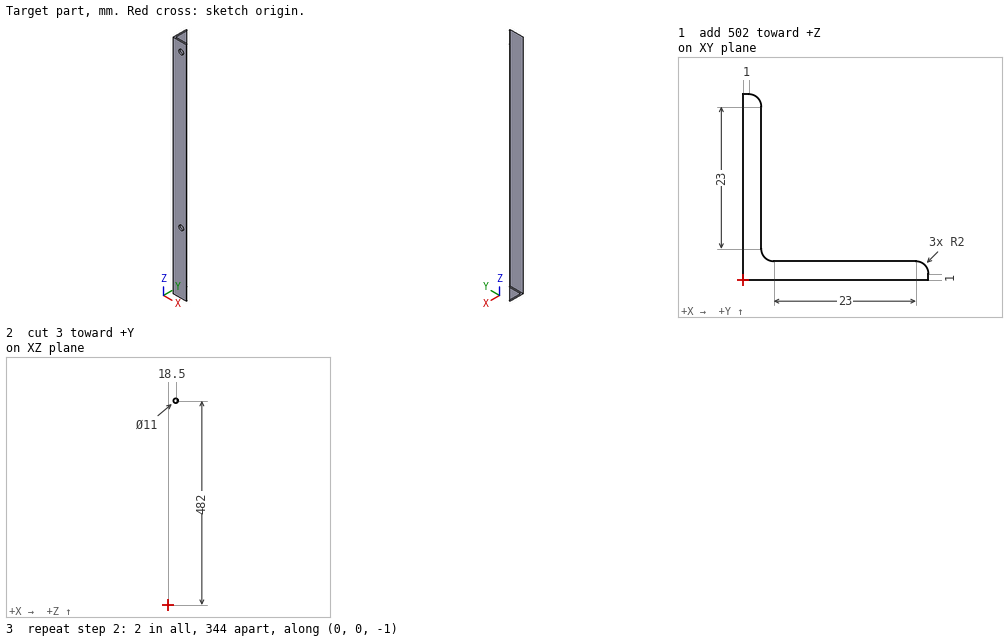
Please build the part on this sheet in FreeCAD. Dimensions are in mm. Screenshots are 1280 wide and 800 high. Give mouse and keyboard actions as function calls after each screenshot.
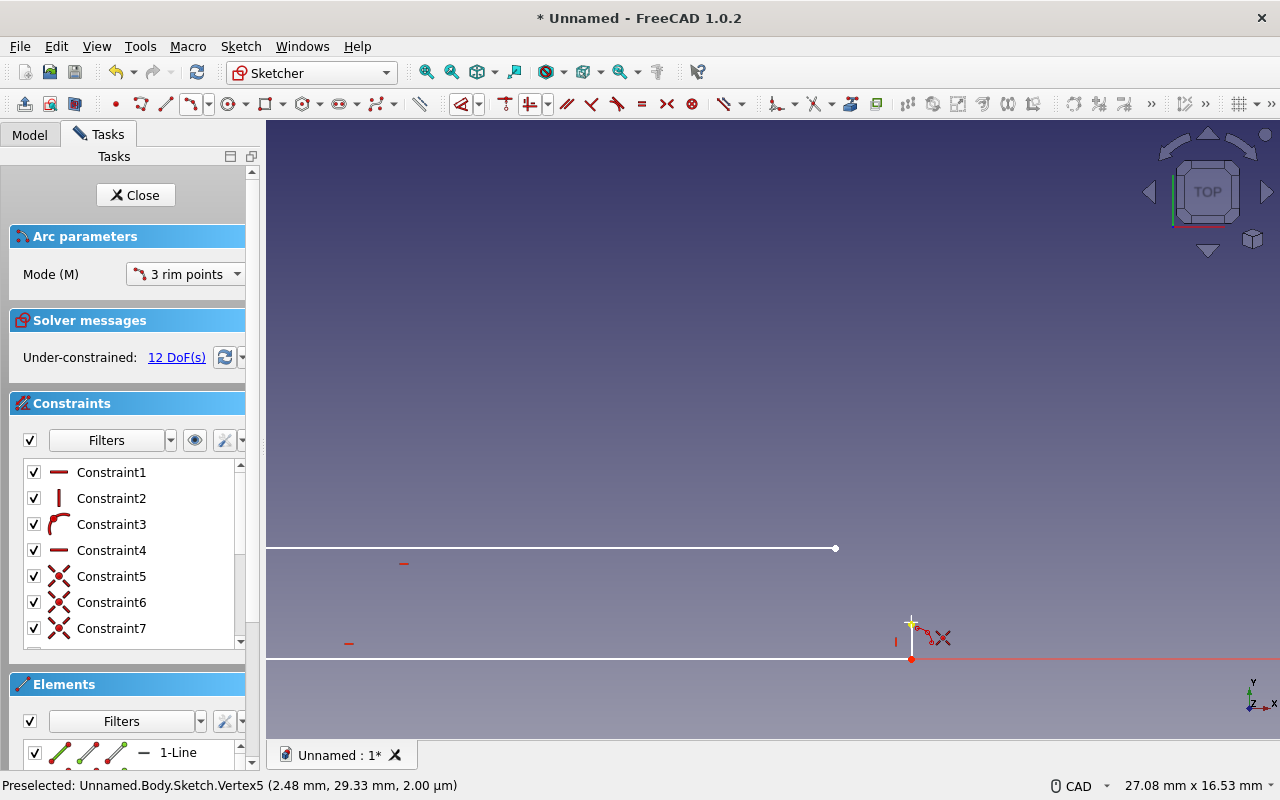
click(912, 625)
click(836, 548)
click(889, 569)
key(Escape)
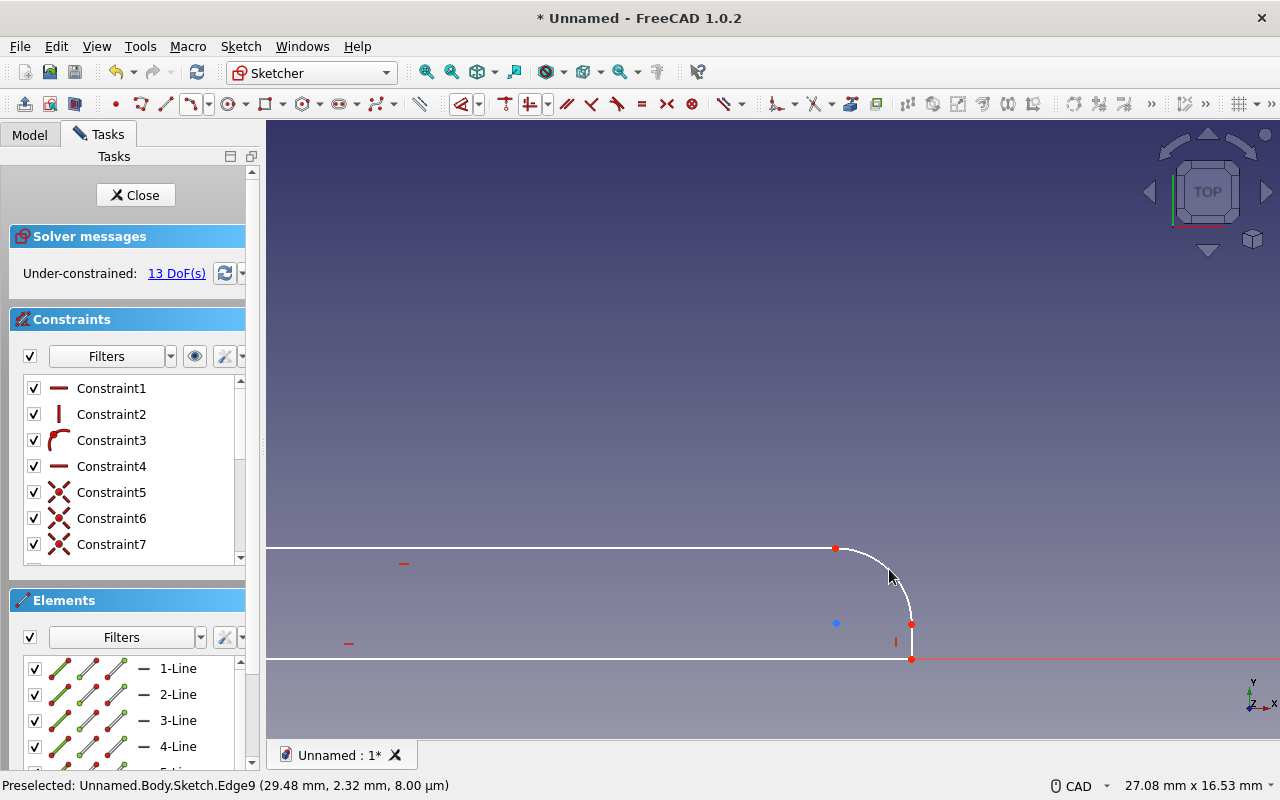
click(577, 548)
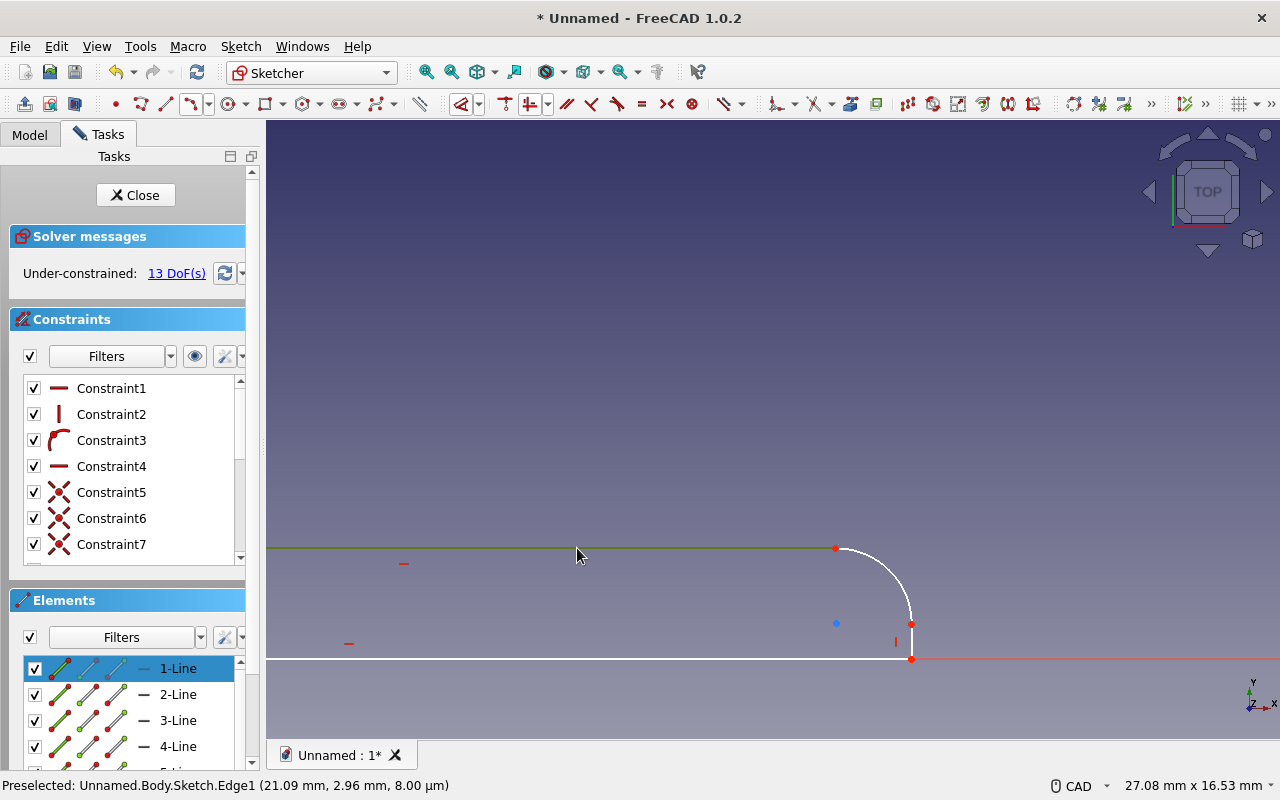
scroll(911, 623, down, 5)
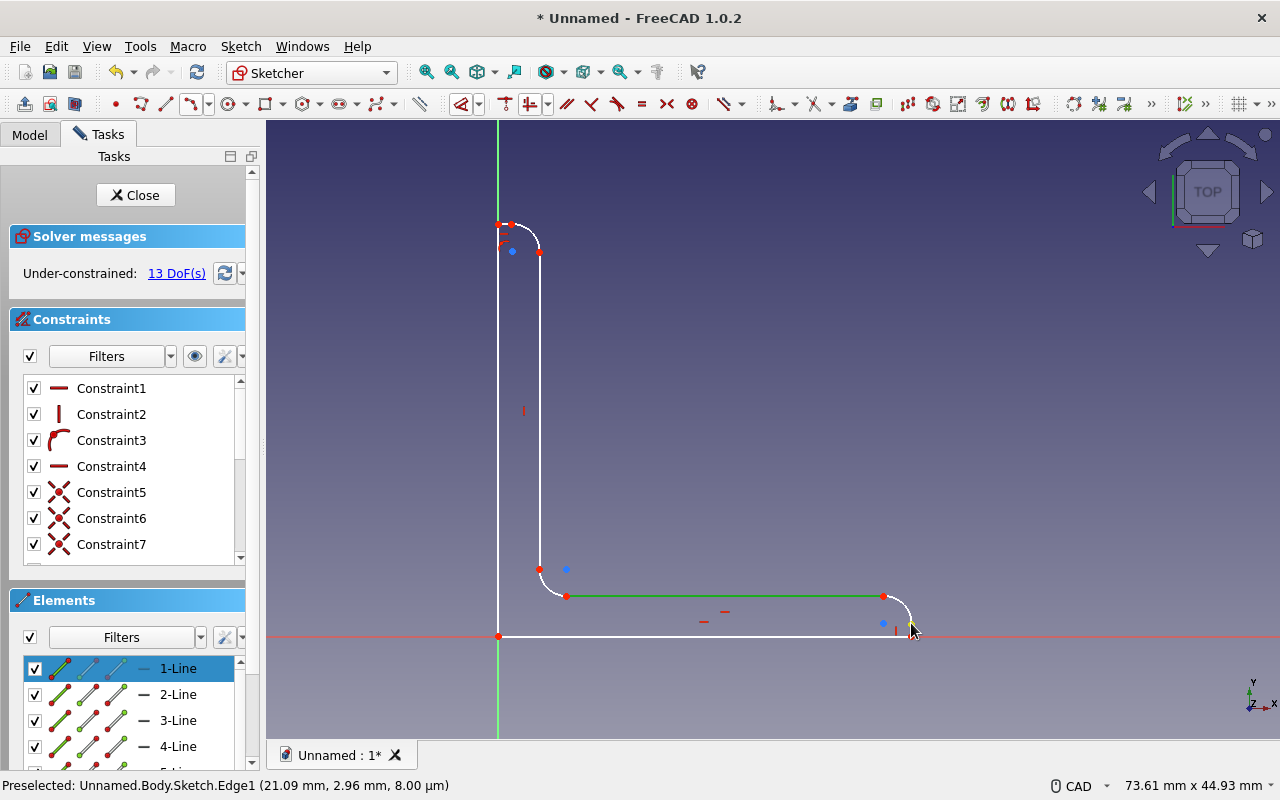
click(543, 581)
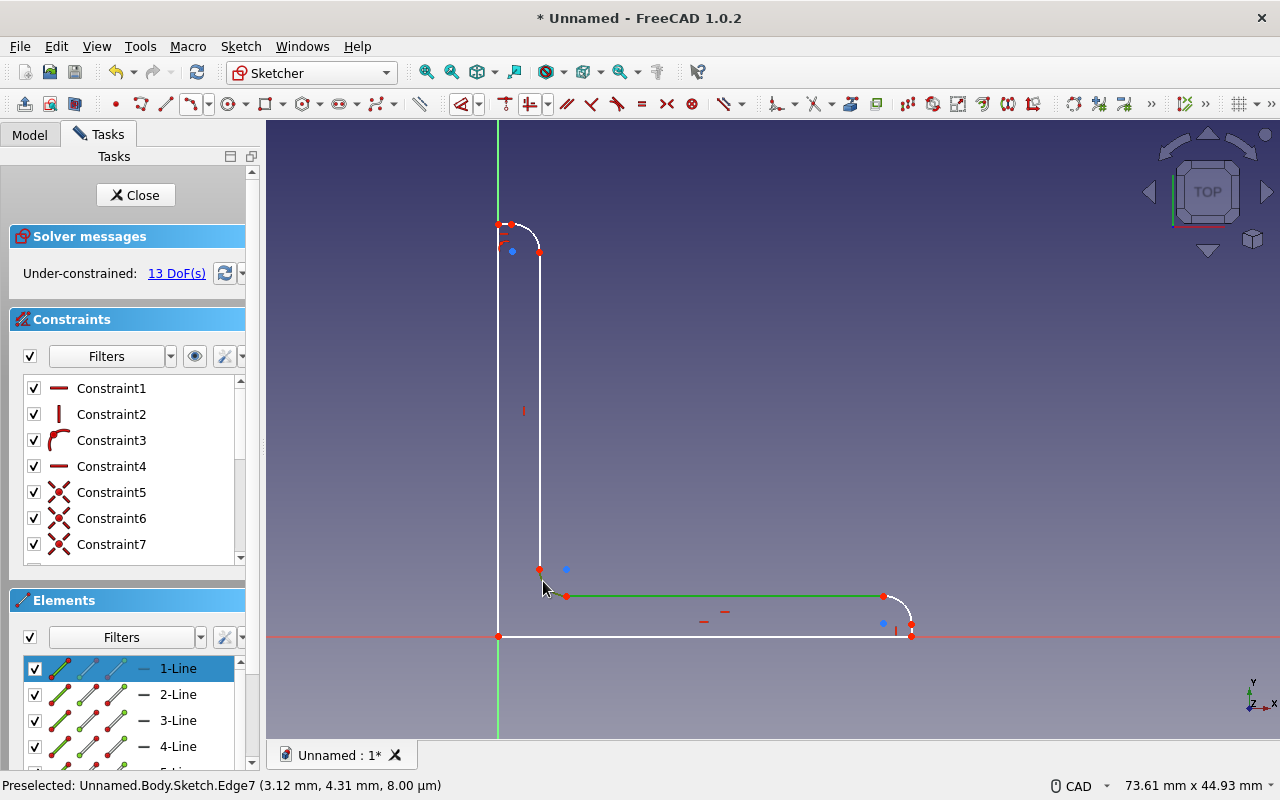
click(617, 104)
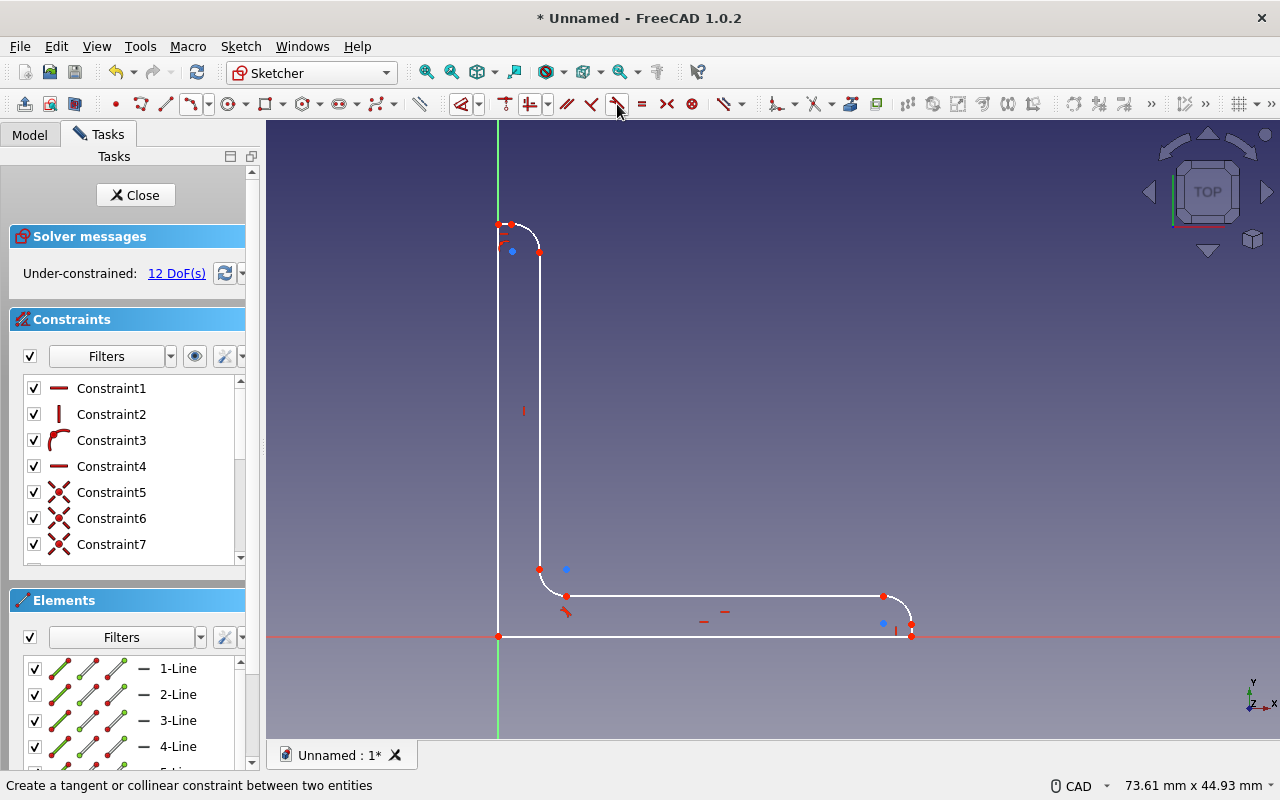
click(789, 596)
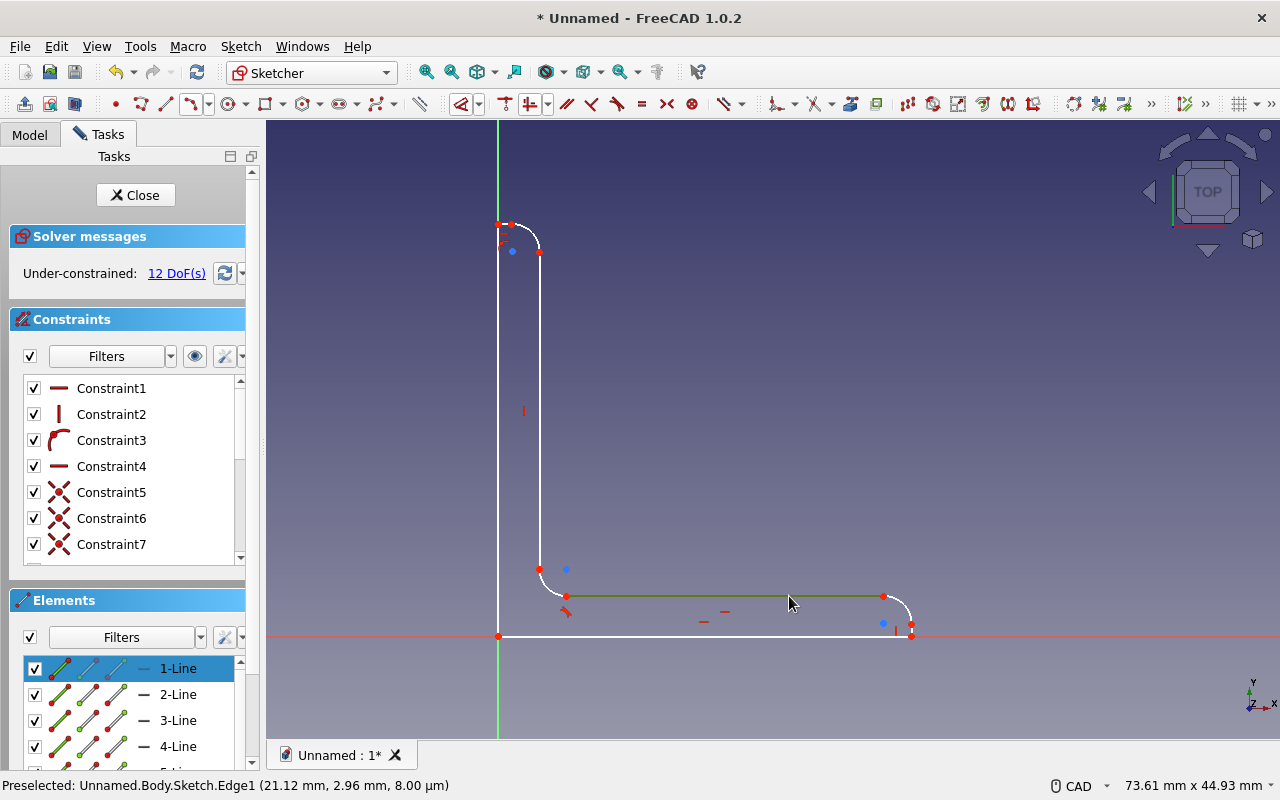
click(909, 611)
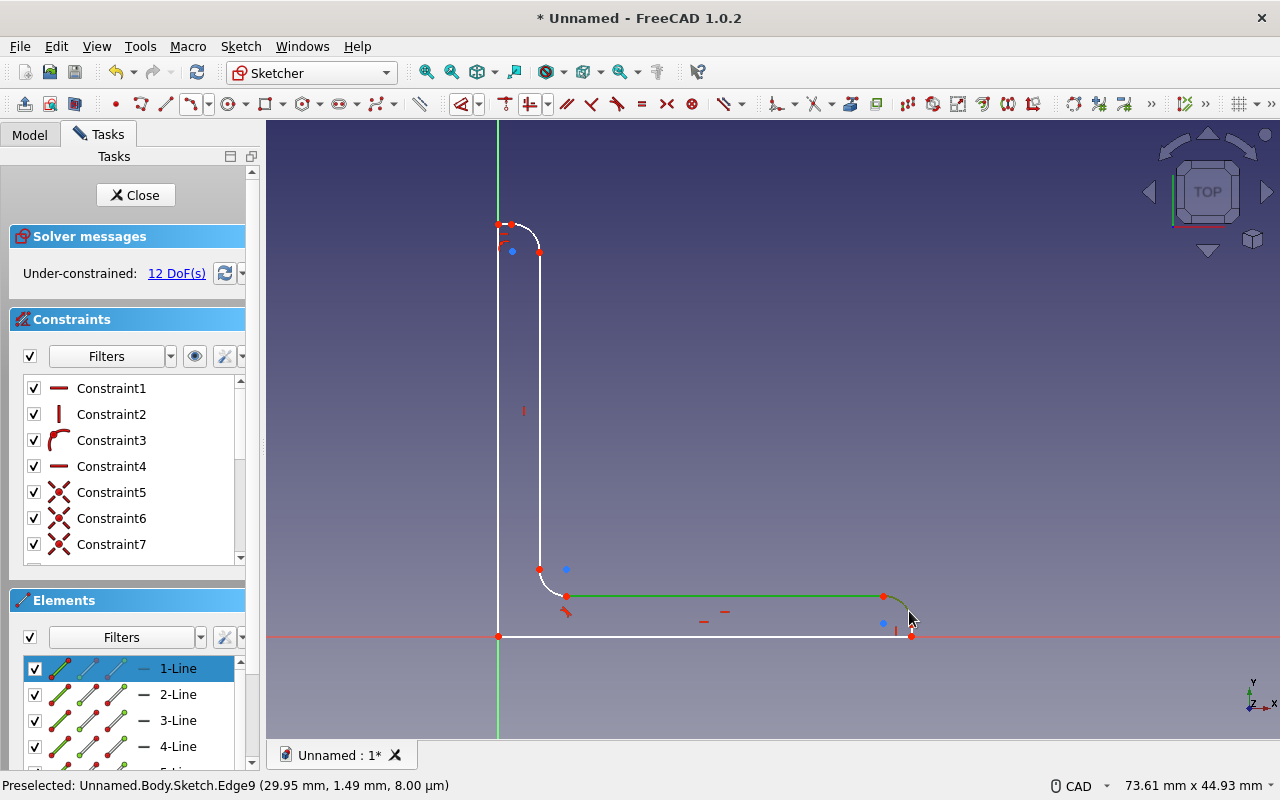
click(617, 104)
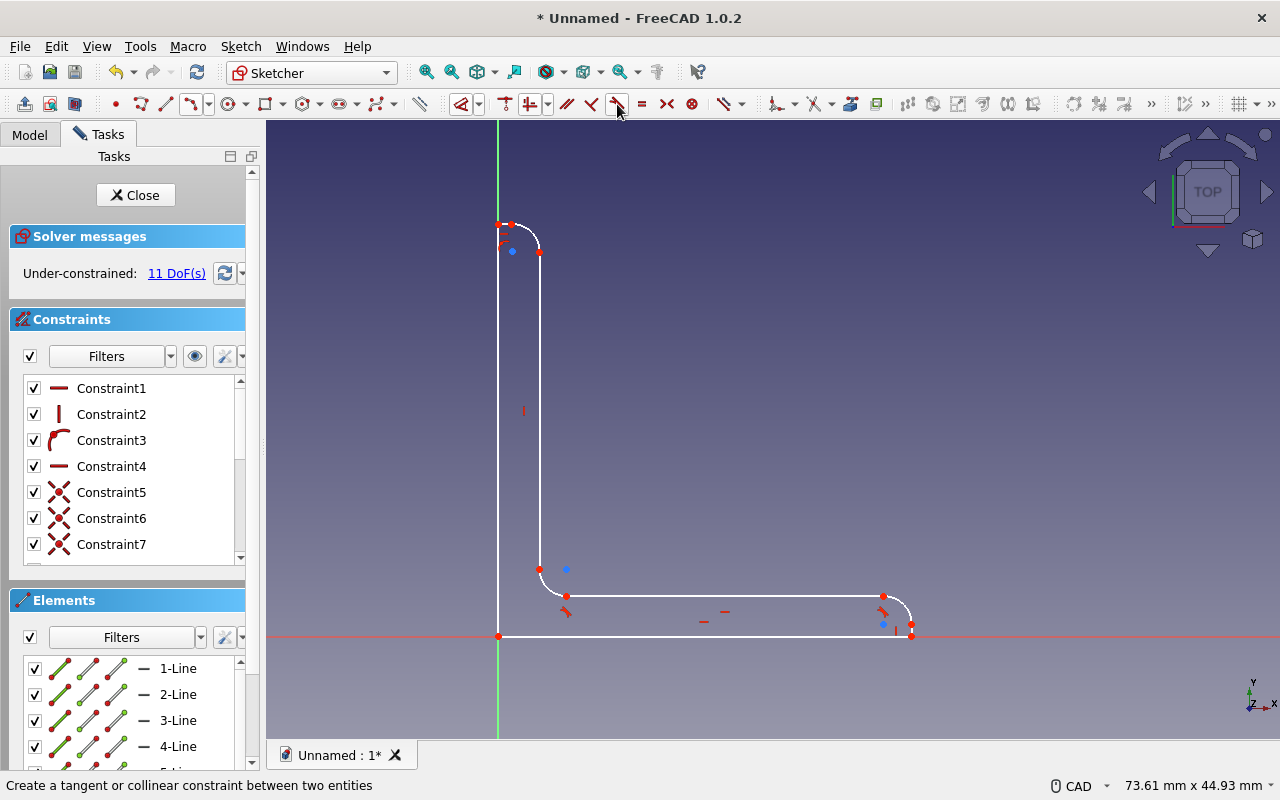
click(540, 474)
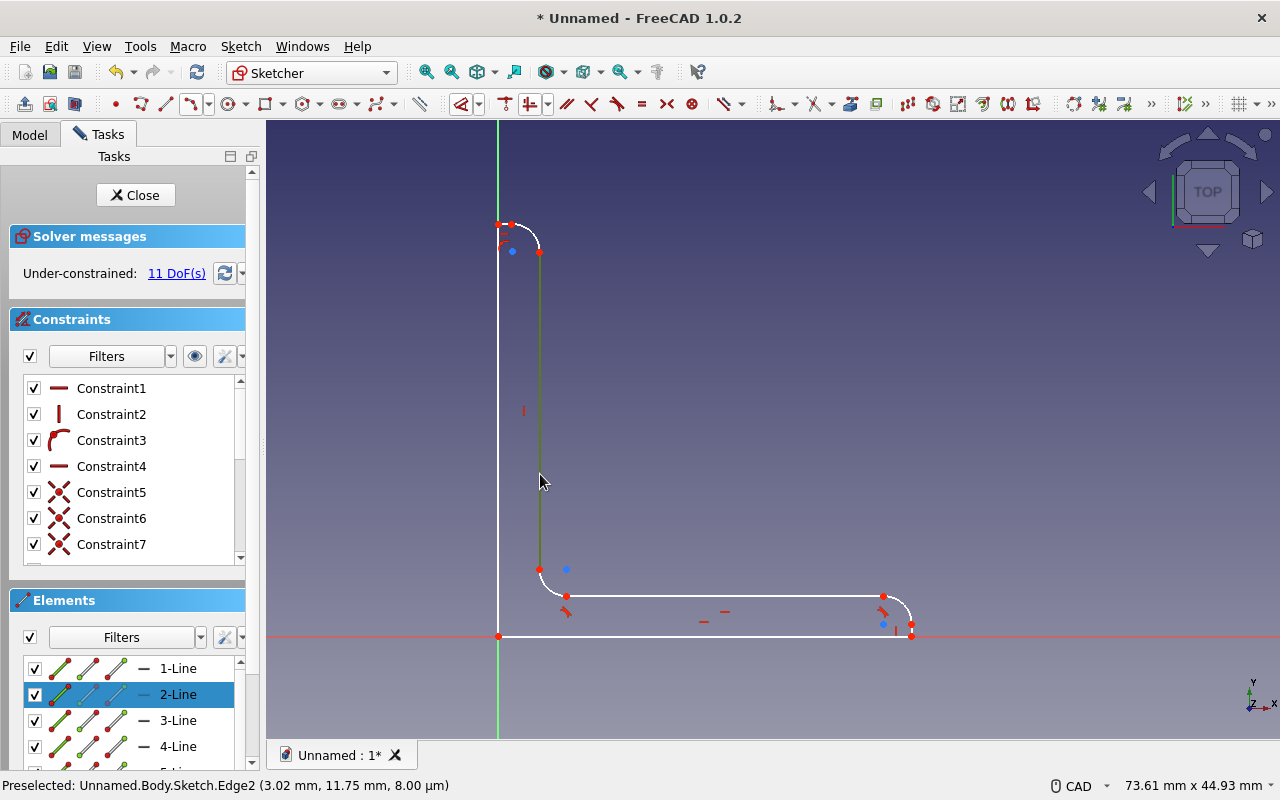
click(543, 581)